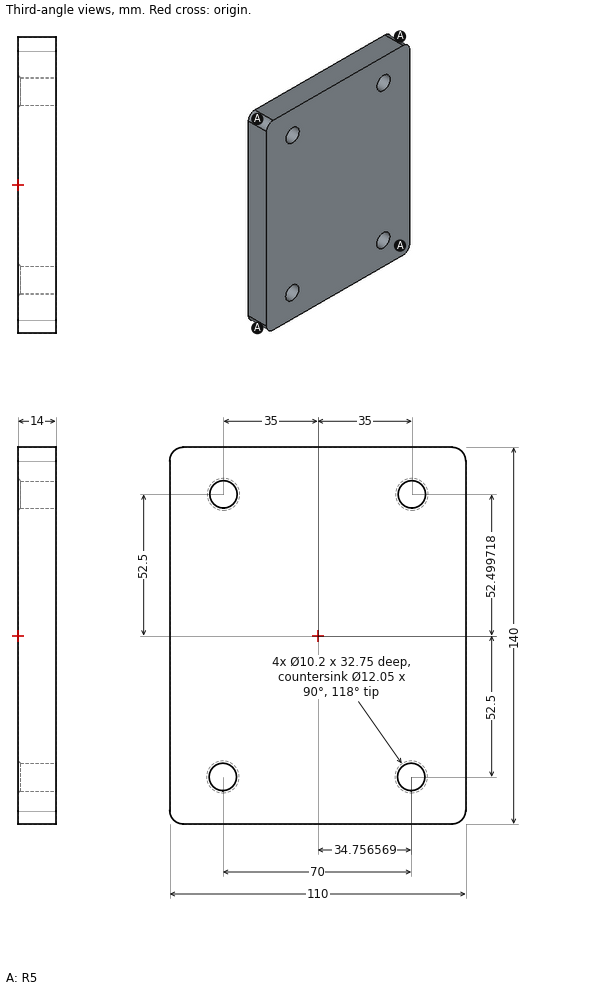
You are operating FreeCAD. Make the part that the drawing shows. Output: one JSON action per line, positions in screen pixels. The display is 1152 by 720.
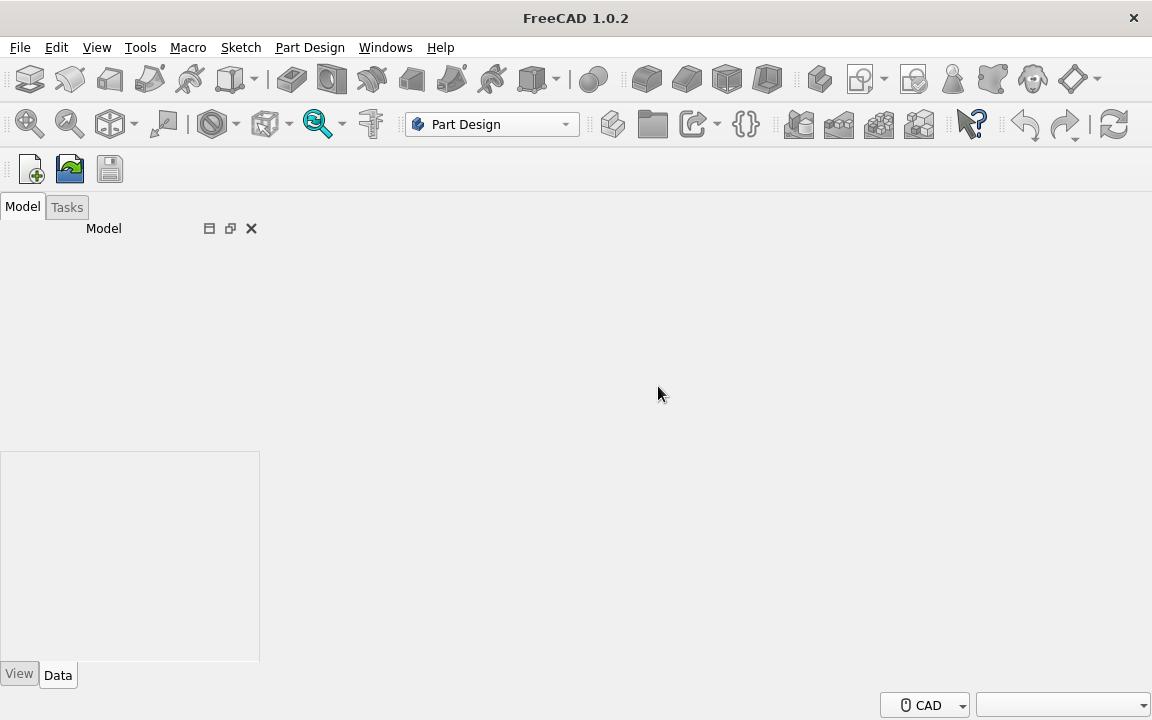
{"action": "left_click", "coordinate": [30, 170]}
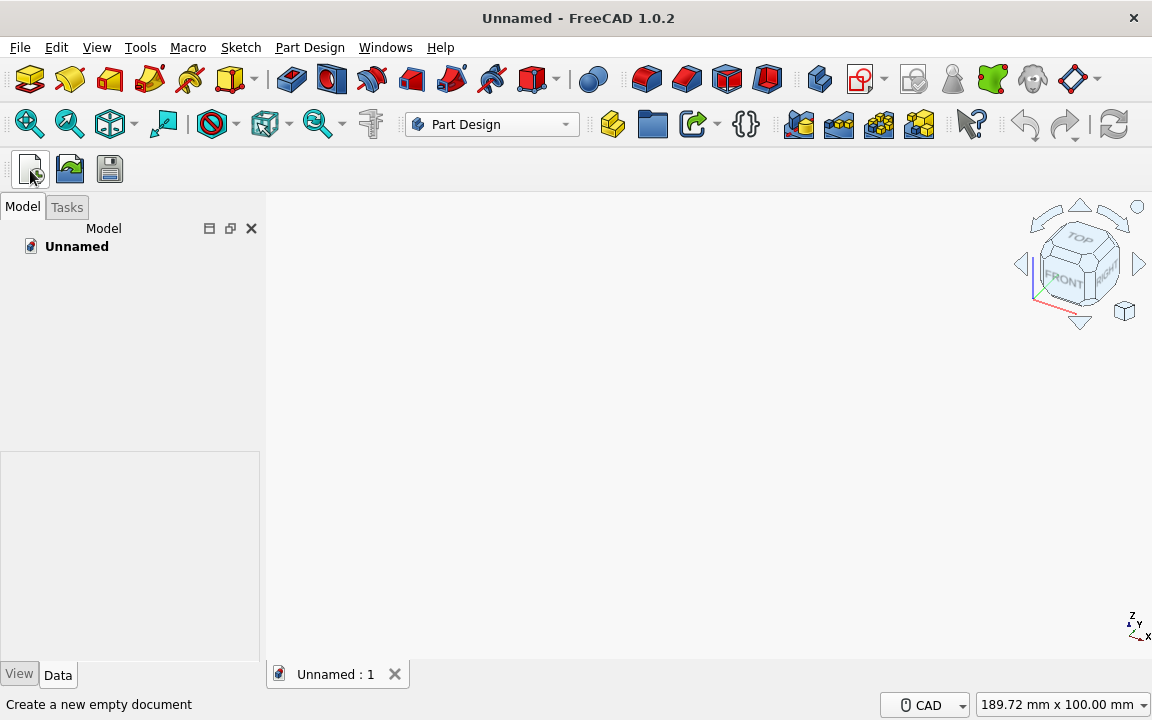
{"action": "left_click", "coordinate": [860, 80]}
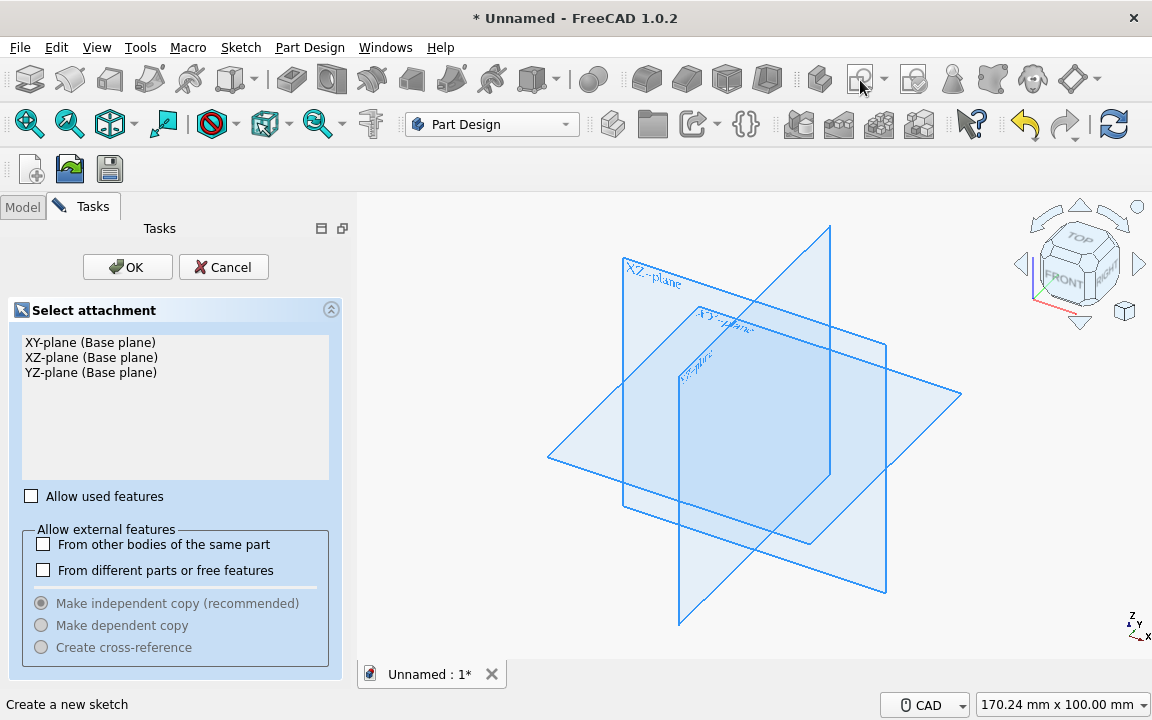
{"action": "left_click", "coordinate": [82, 372]}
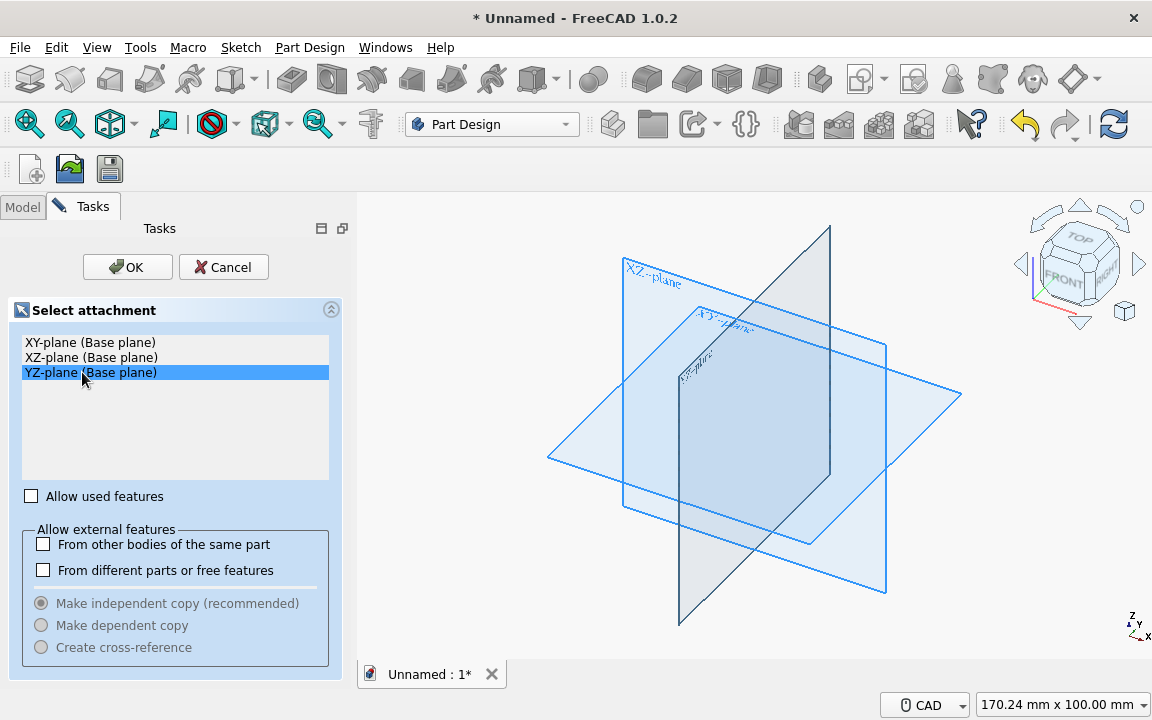
{"action": "left_click", "coordinate": [128, 267]}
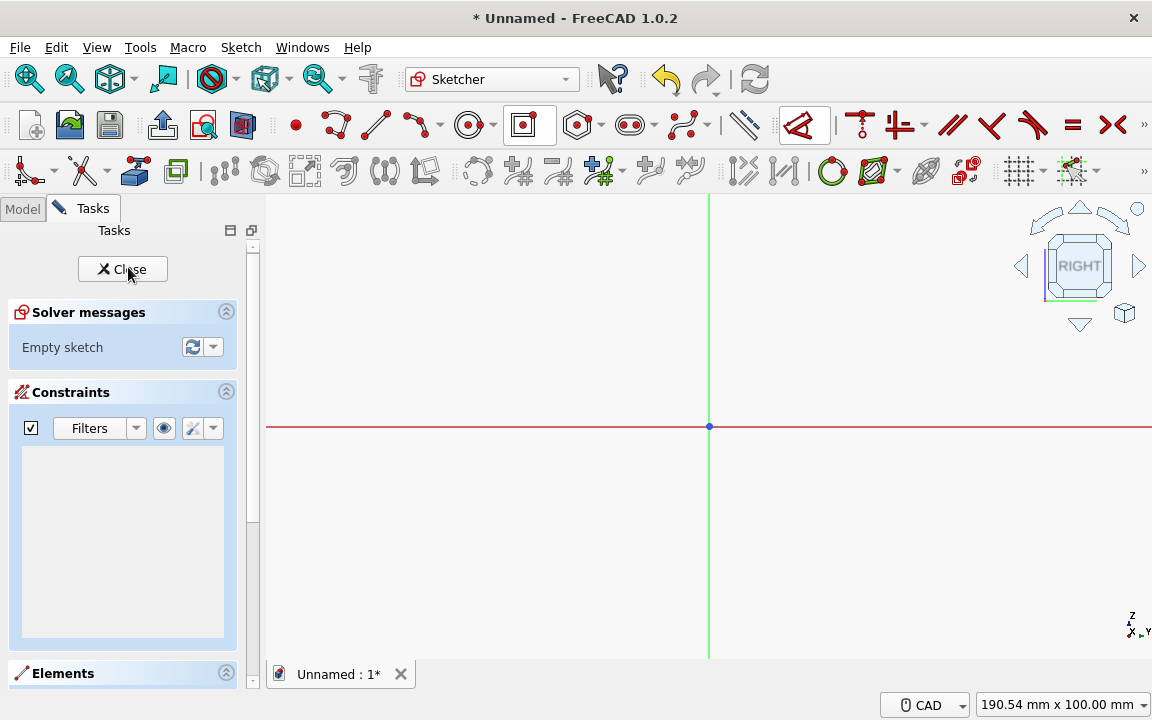
{"action": "scroll", "coordinate": [585, 426], "scroll_direction": "down", "scroll_amount": 4}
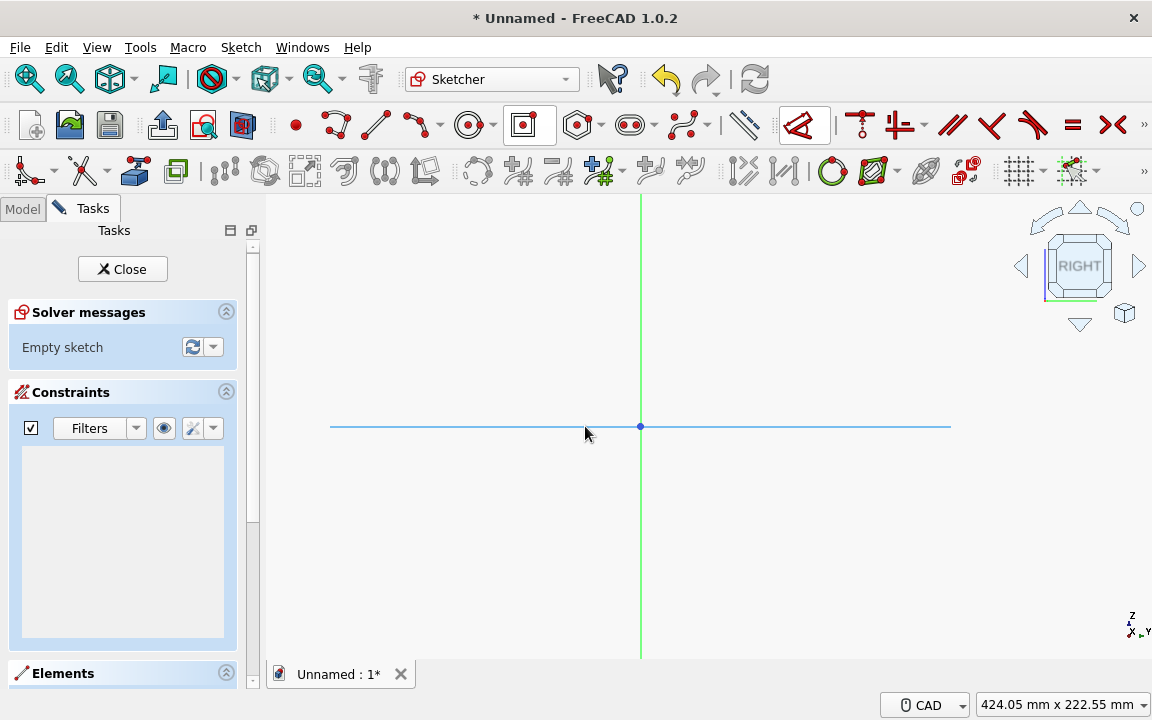
{"action": "left_click", "coordinate": [524, 126]}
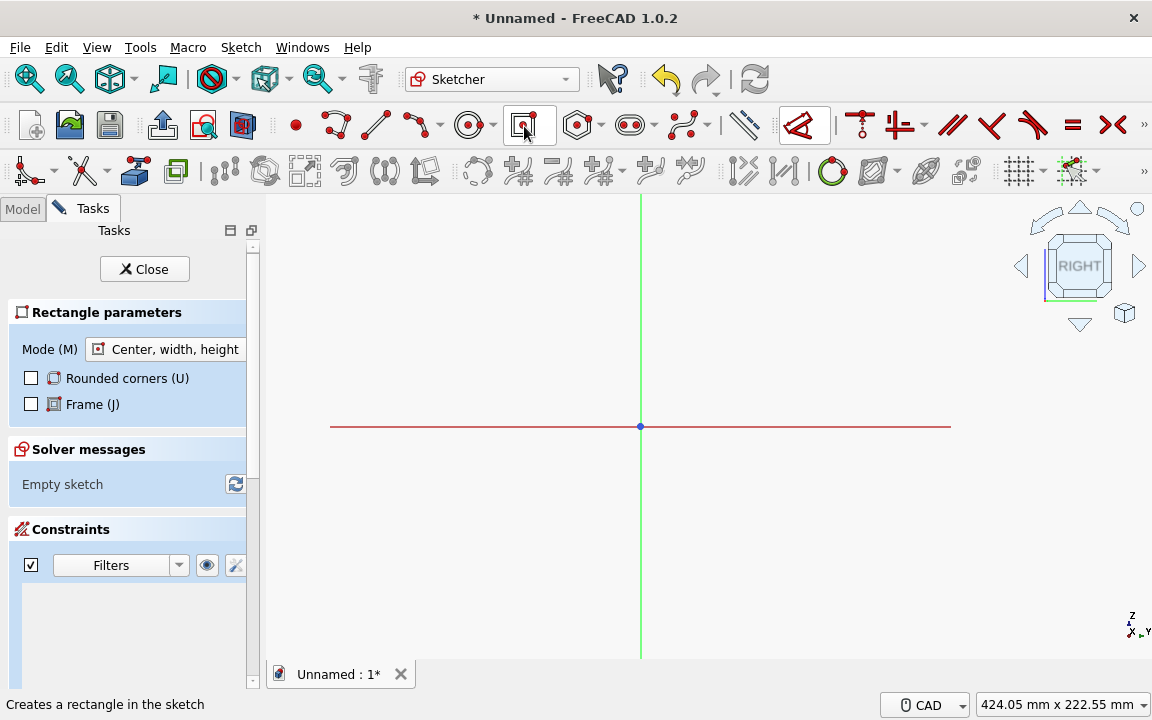
{"action": "left_click", "coordinate": [641, 426]}
{"action": "left_click", "coordinate": [756, 280]}
{"action": "key", "text": "Escape"}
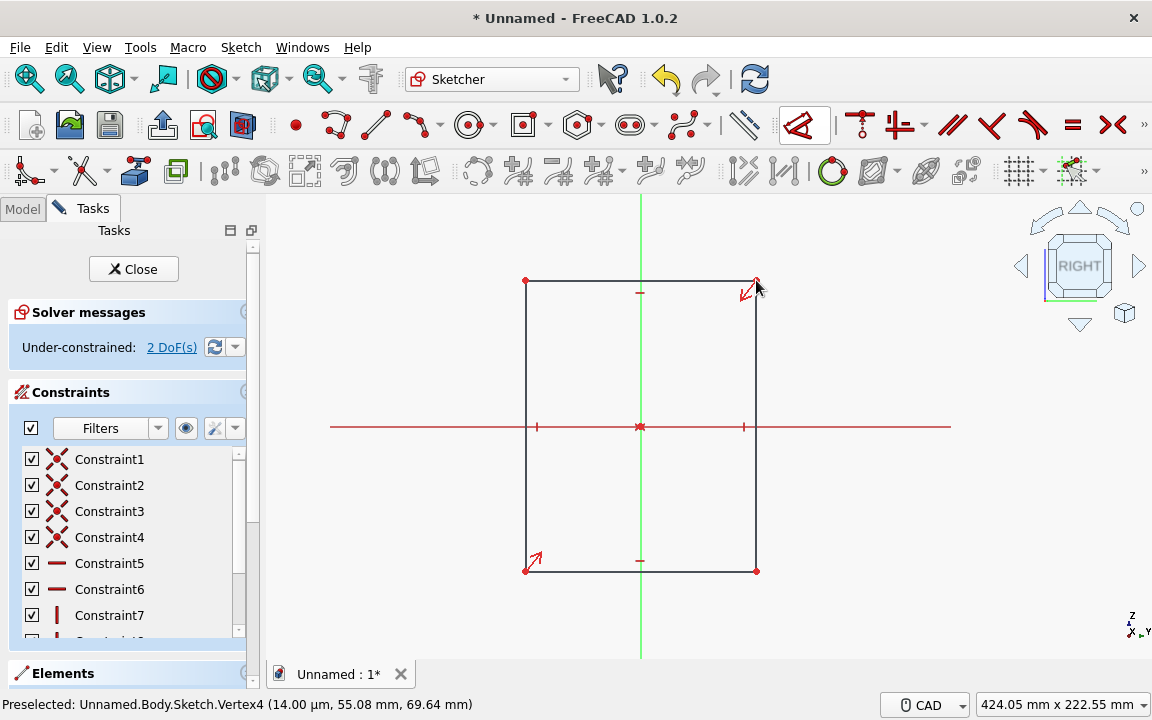
{"action": "left_click", "coordinate": [798, 126]}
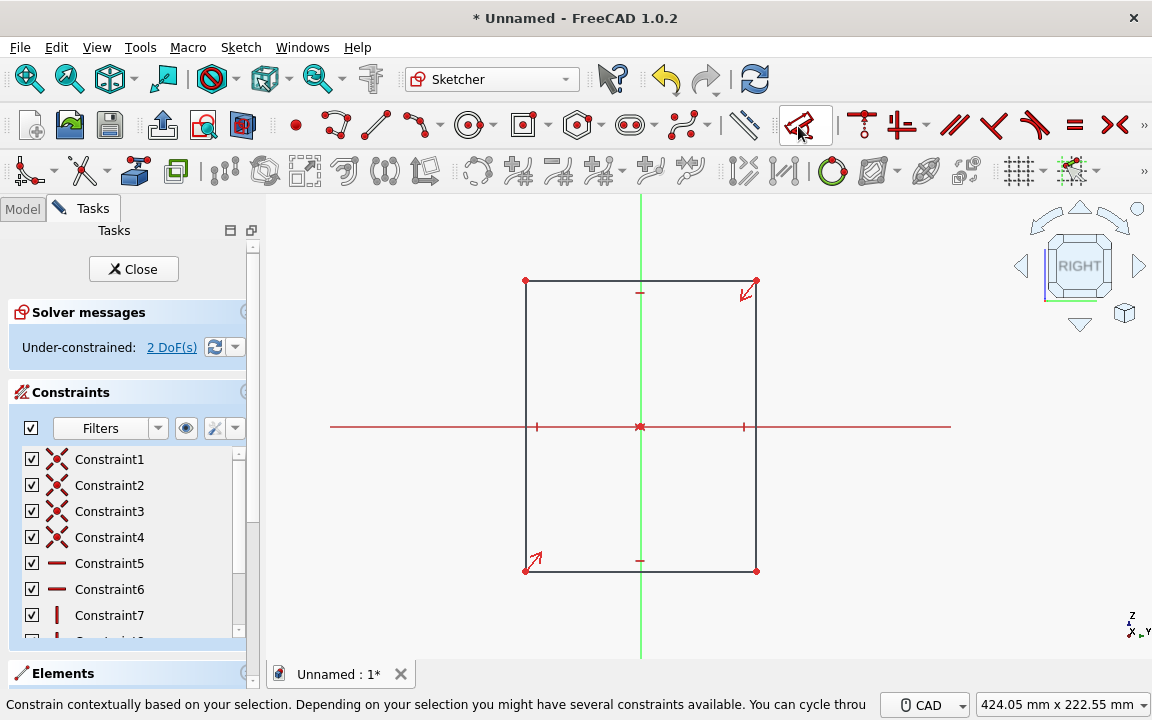
{"action": "left_click", "coordinate": [595, 572]}
{"action": "left_click", "coordinate": [588, 606]}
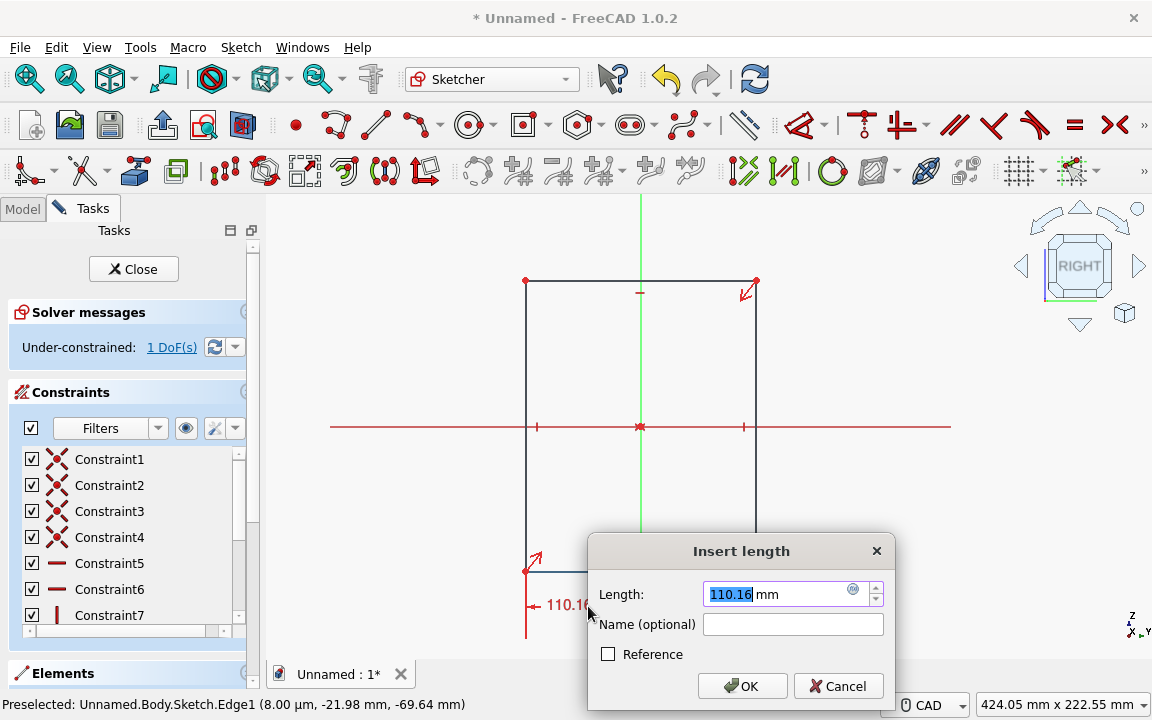
{"action": "type", "text": "110"}
{"action": "key", "text": "Return"}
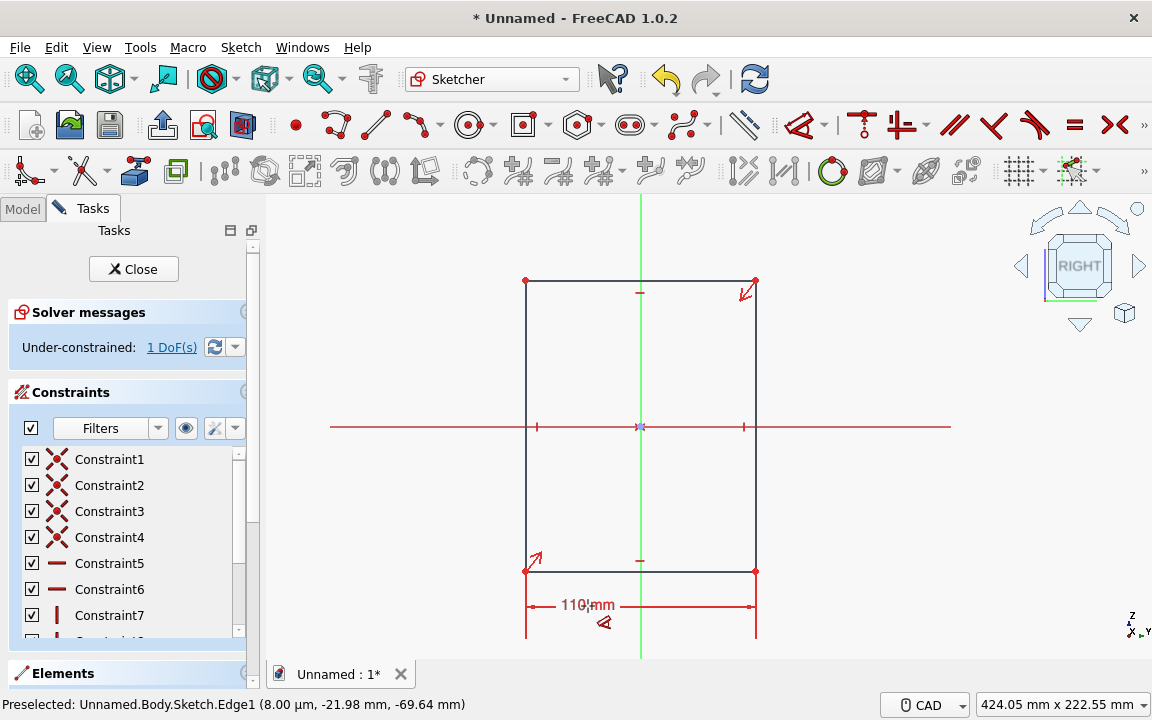
{"action": "left_click", "coordinate": [756, 485]}
{"action": "left_click", "coordinate": [790, 360]}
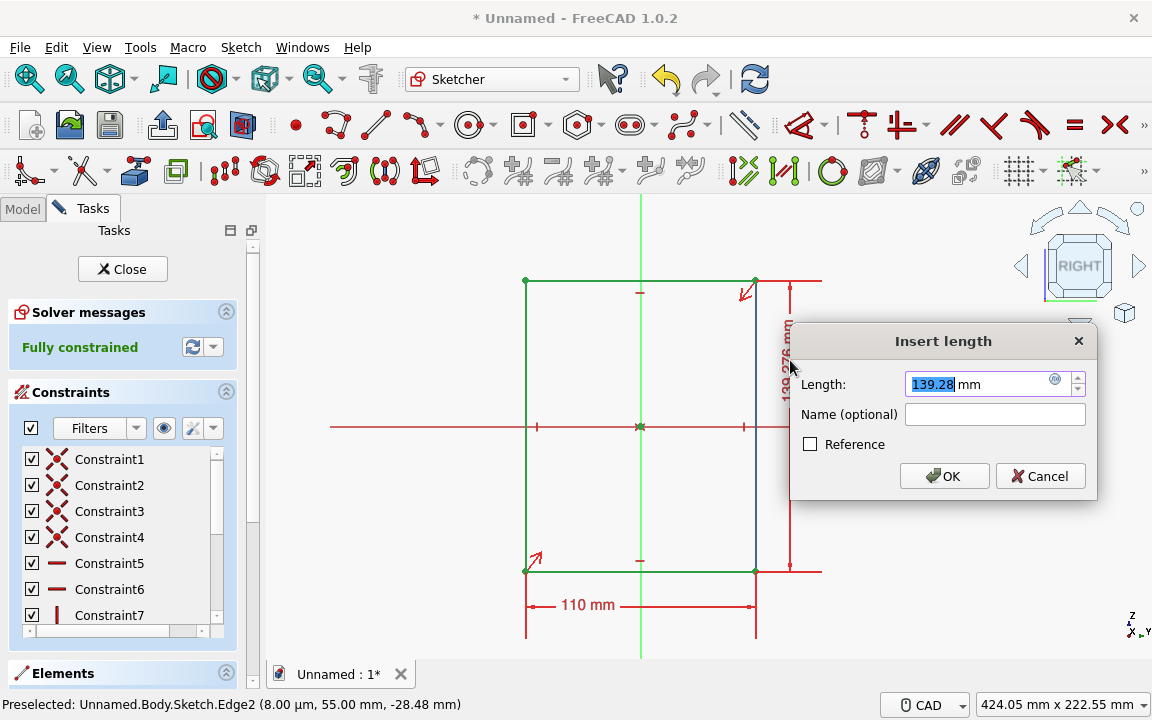
{"action": "type", "text": "140"}
{"action": "key", "text": "Return"}
{"action": "key", "text": "Escape"}